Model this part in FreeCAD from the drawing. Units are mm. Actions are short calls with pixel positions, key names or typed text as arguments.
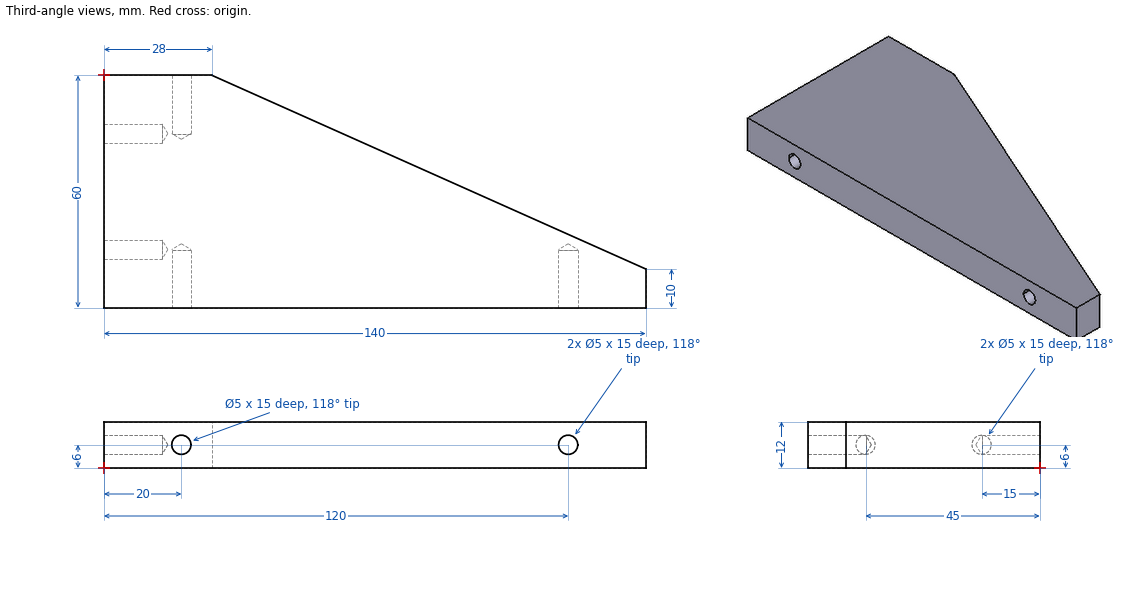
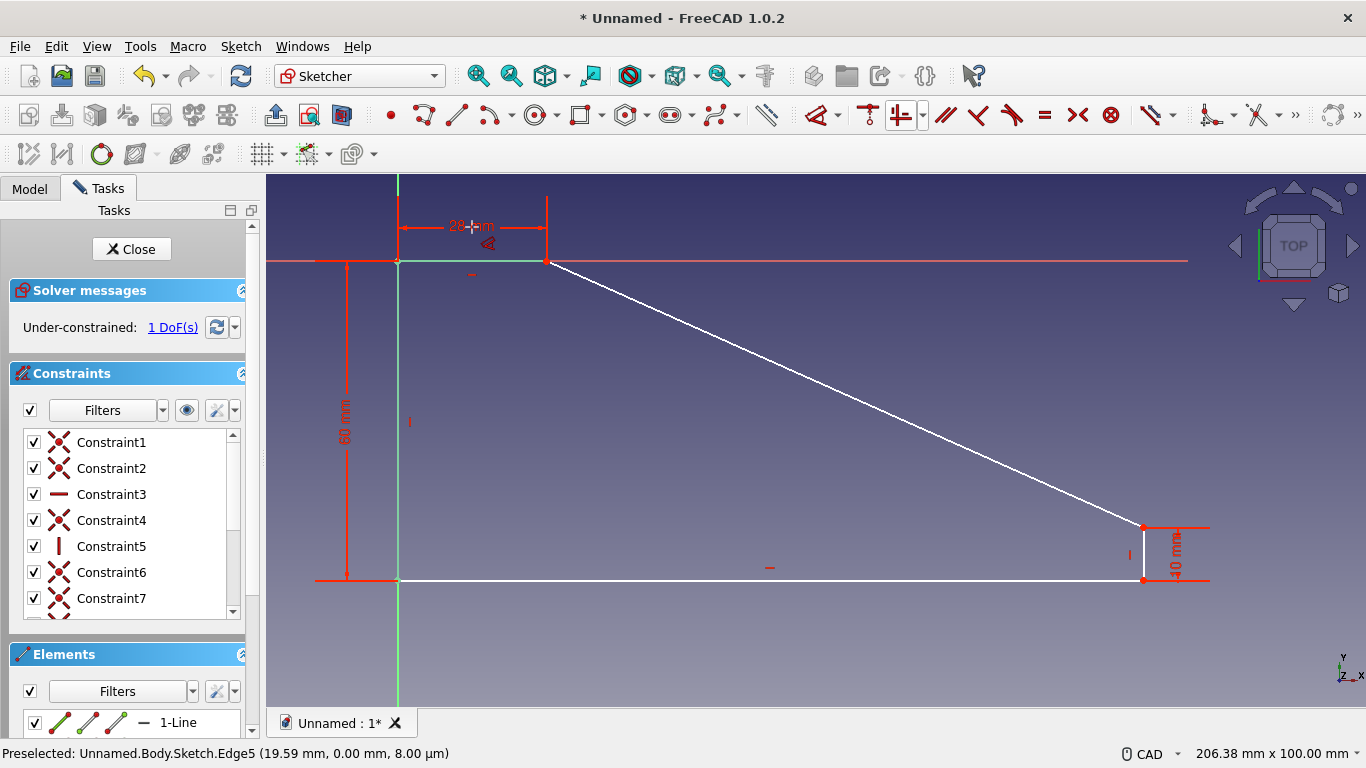
click(621, 581)
click(771, 615)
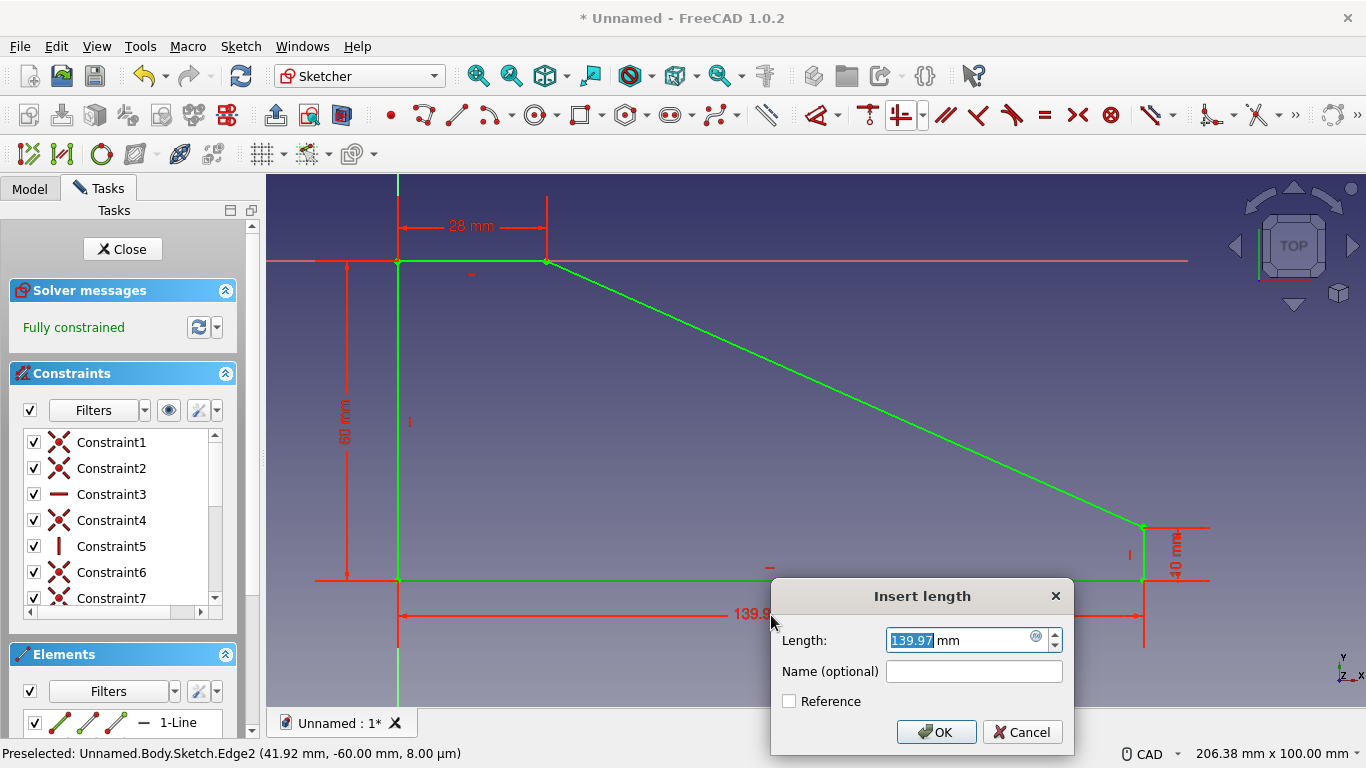
text(140)
key(Return)
key(Escape)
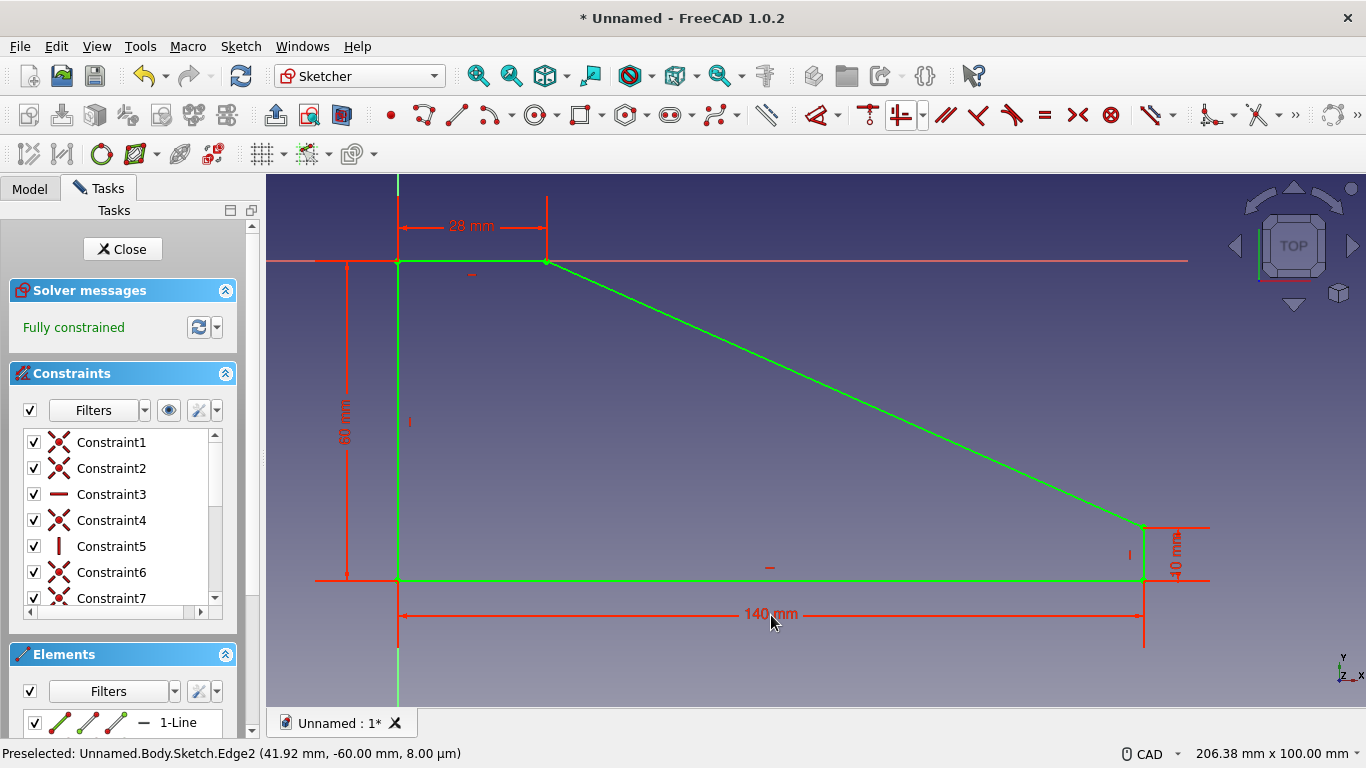
click(123, 249)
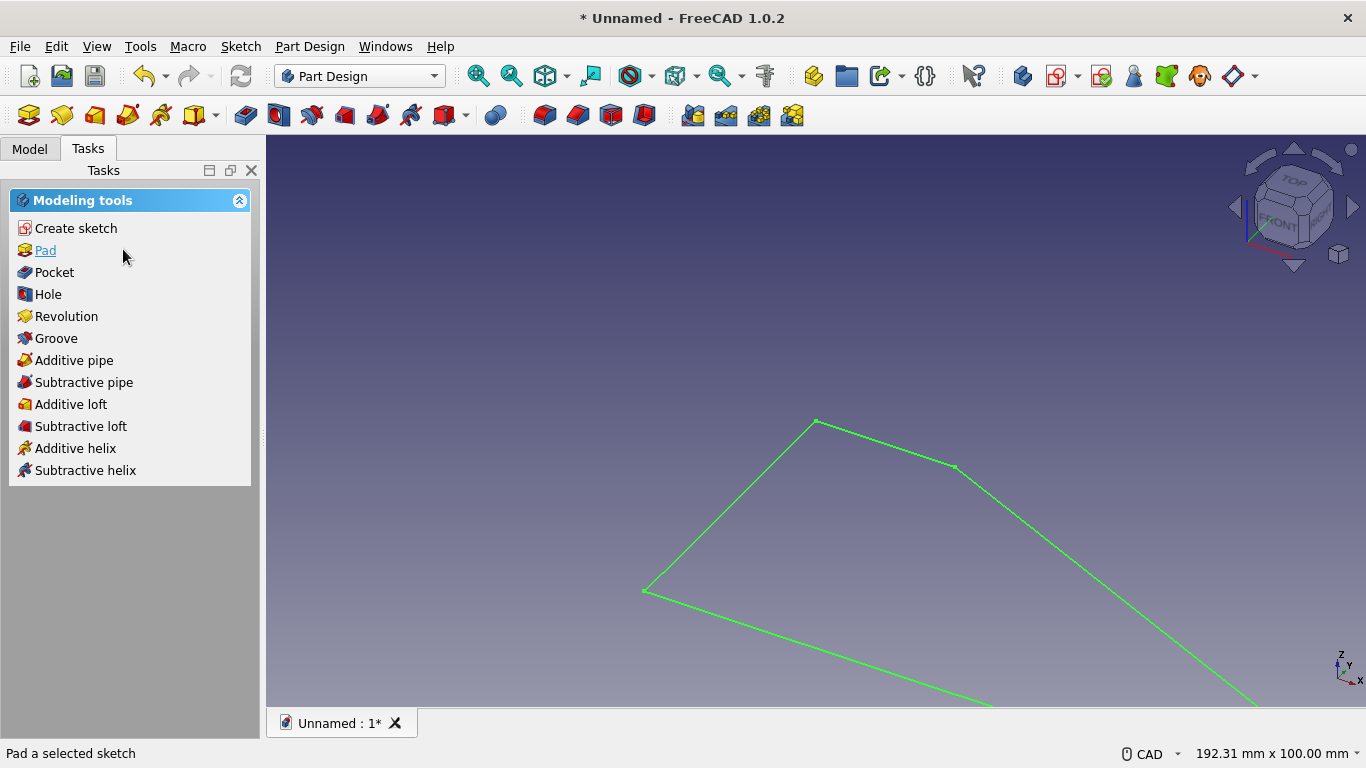
click(29, 116)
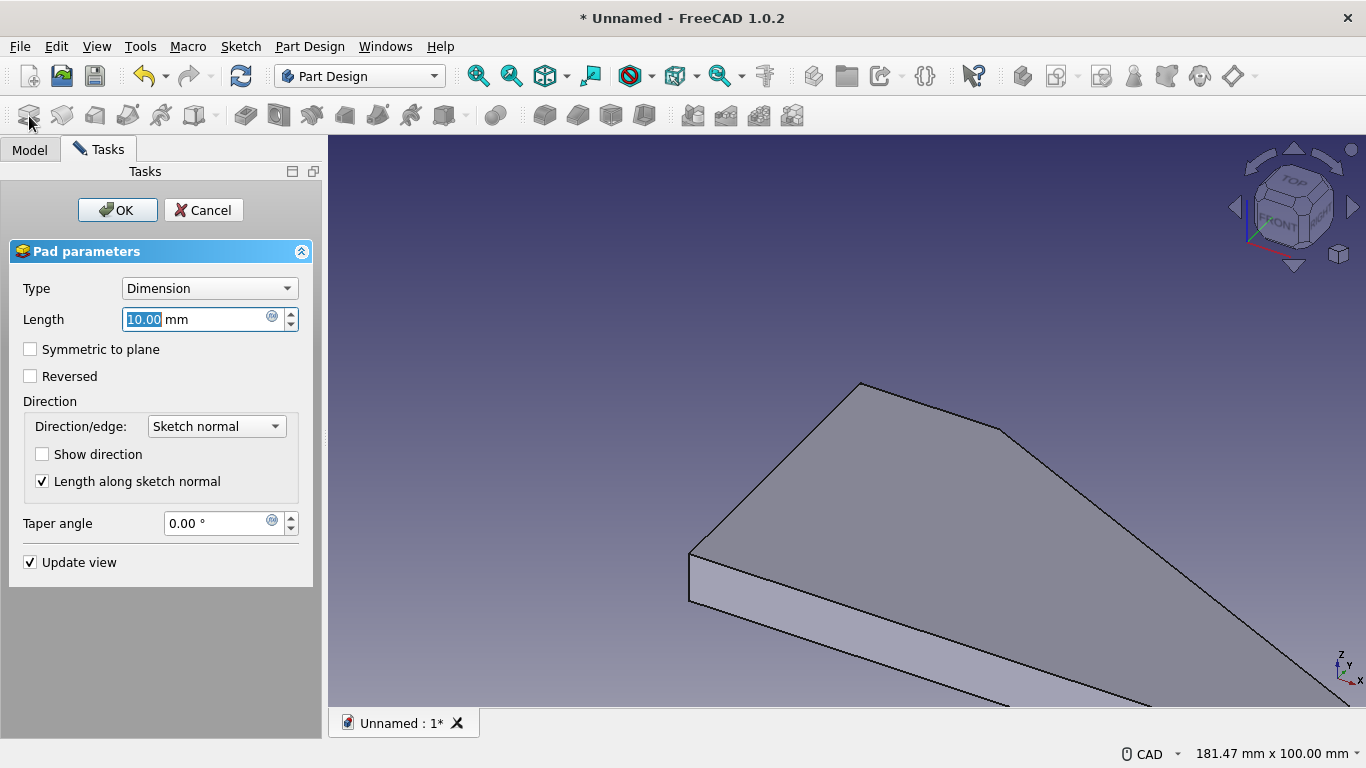
text(12)
key(Tab)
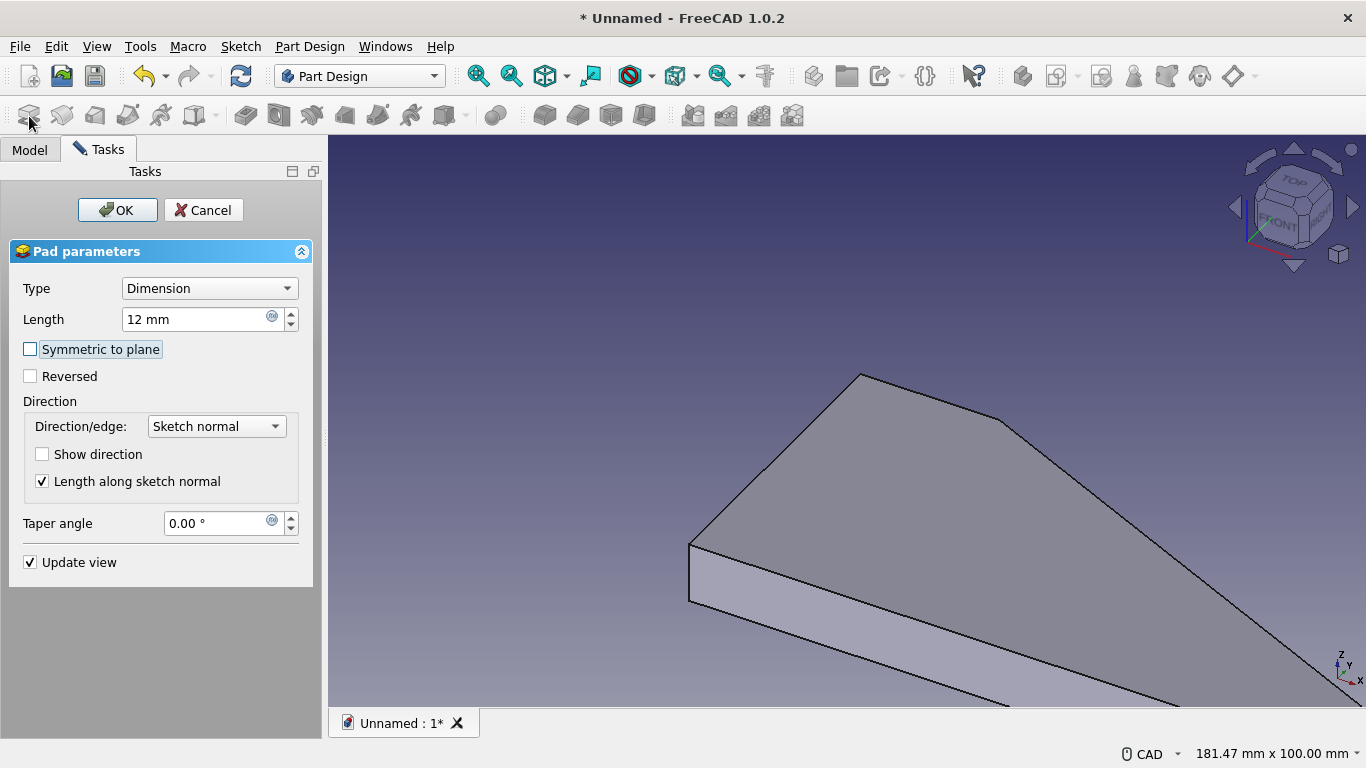
click(118, 210)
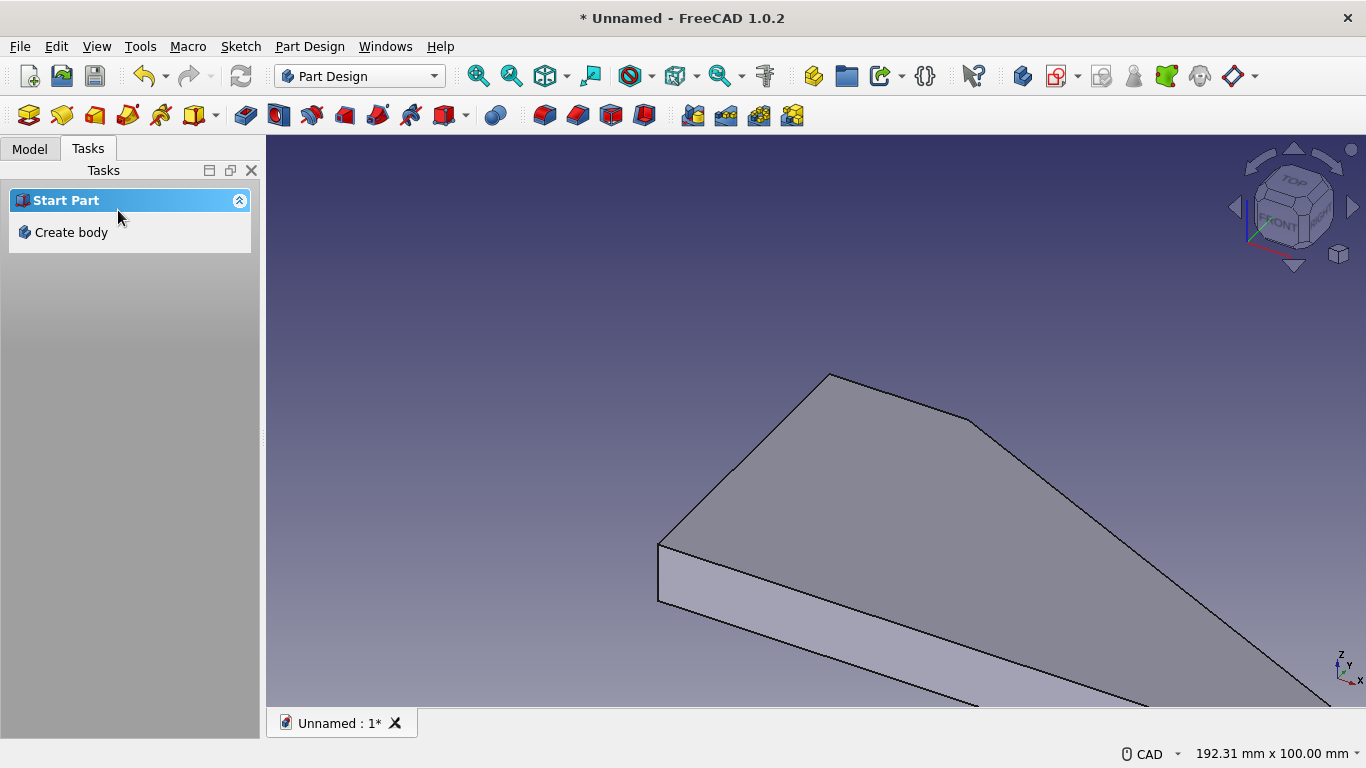
key(v)
key(f)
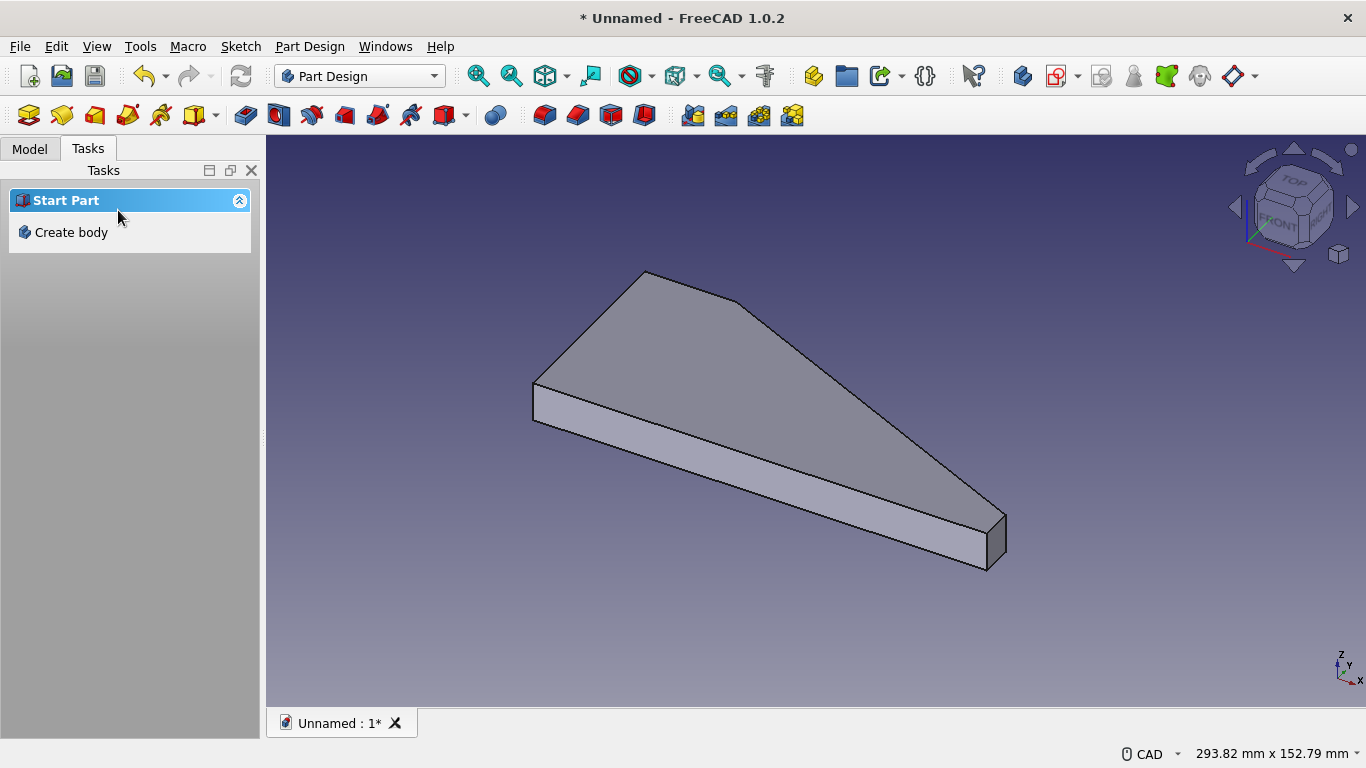
key(6)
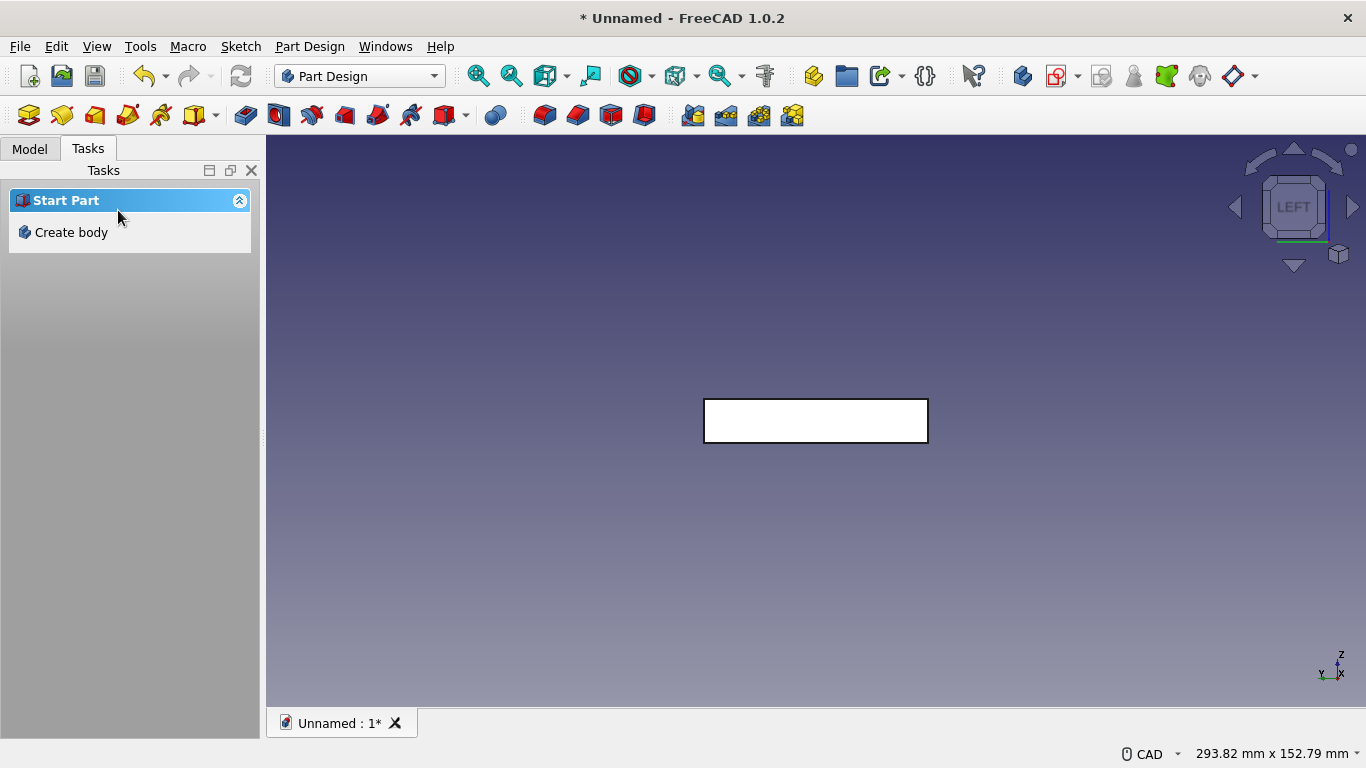
key(v)
key(f)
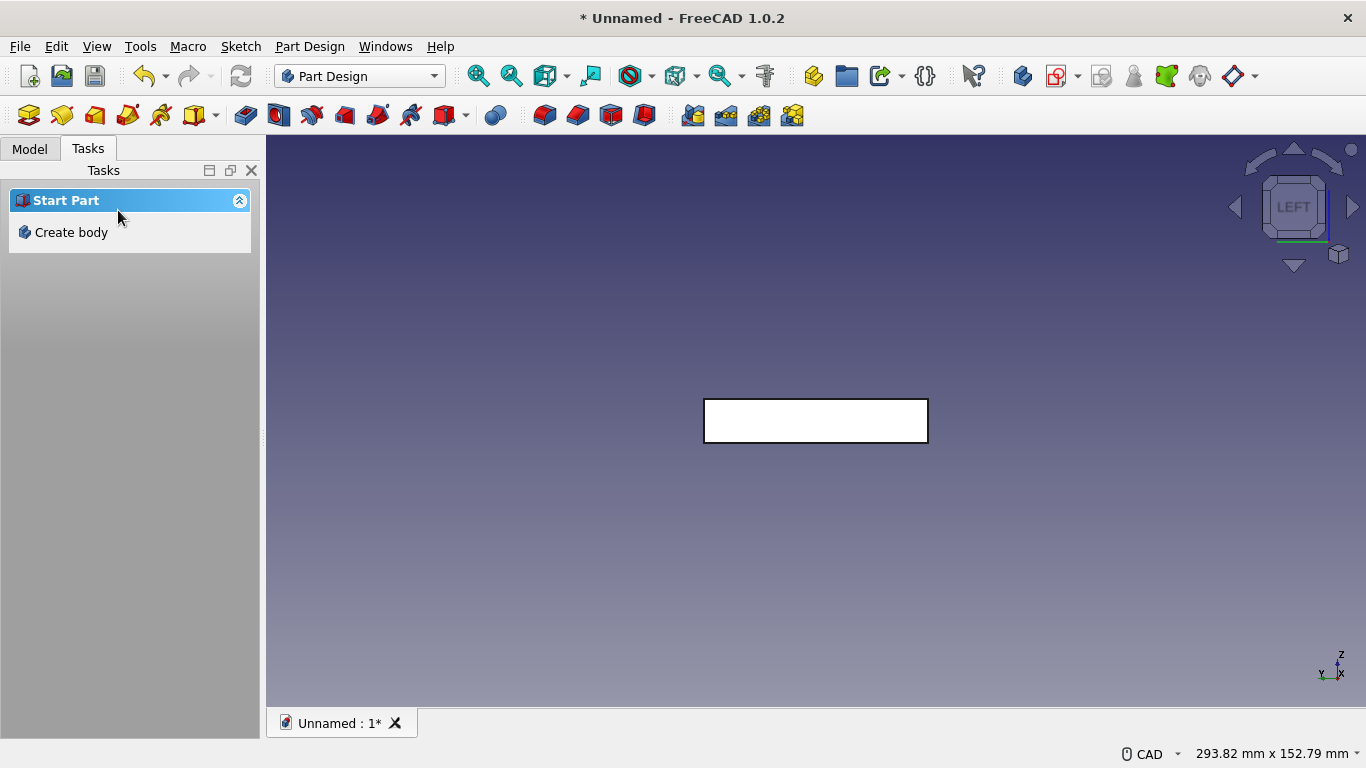
click(752, 420)